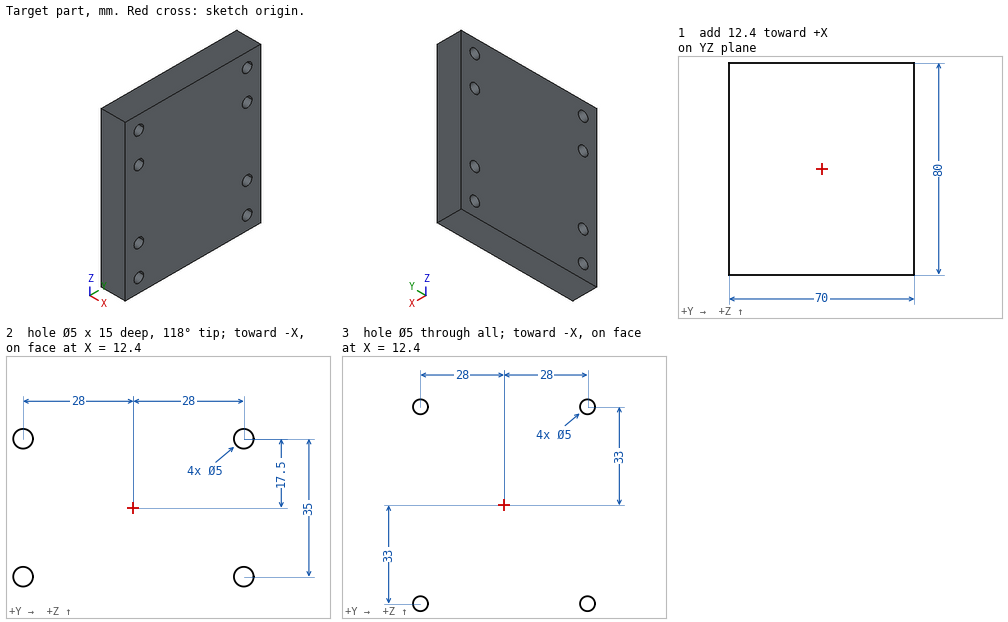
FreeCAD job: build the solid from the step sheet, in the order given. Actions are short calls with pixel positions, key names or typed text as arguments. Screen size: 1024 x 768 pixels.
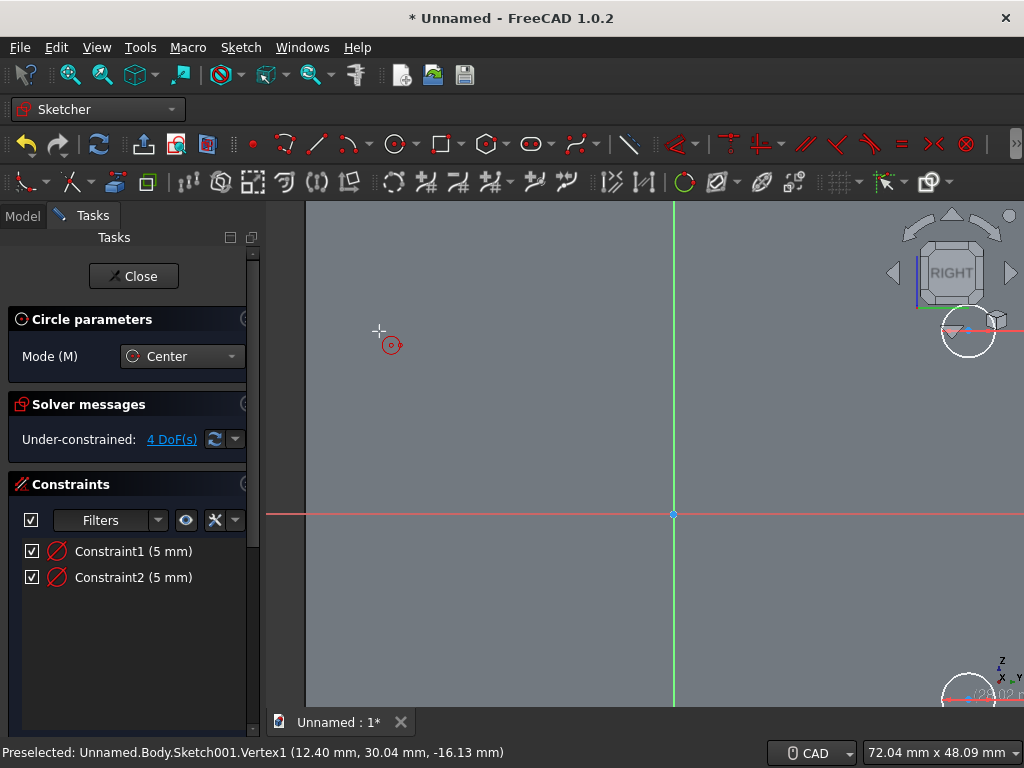
click(379, 330)
move(398, 312)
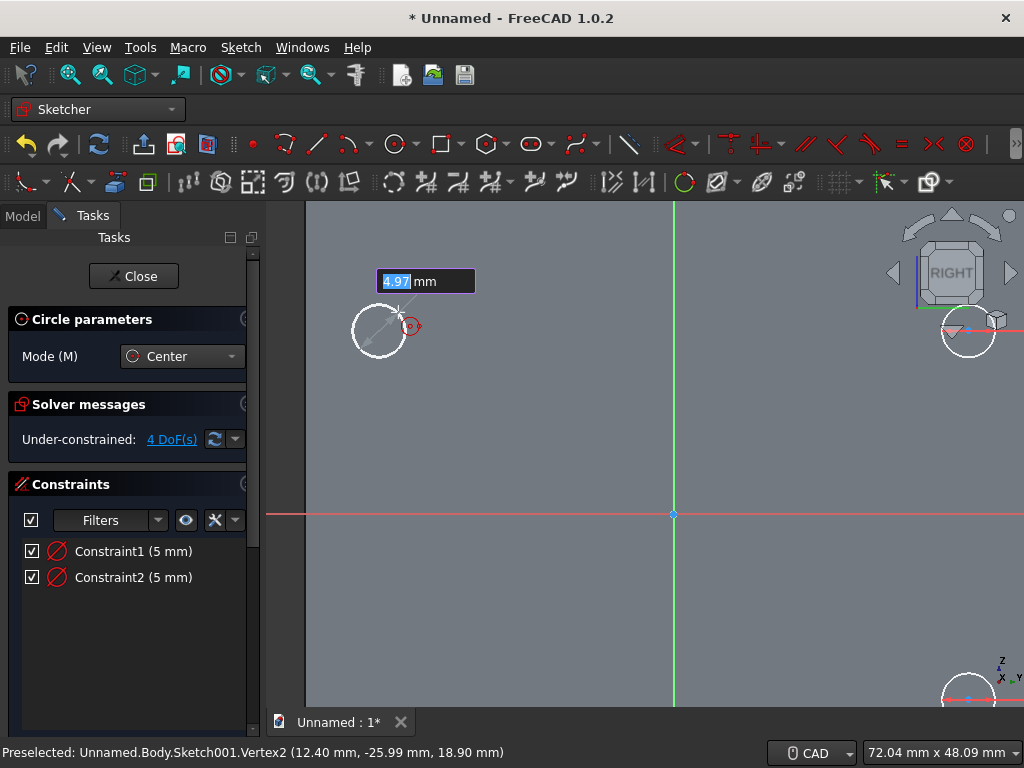
text(5)
key(Return)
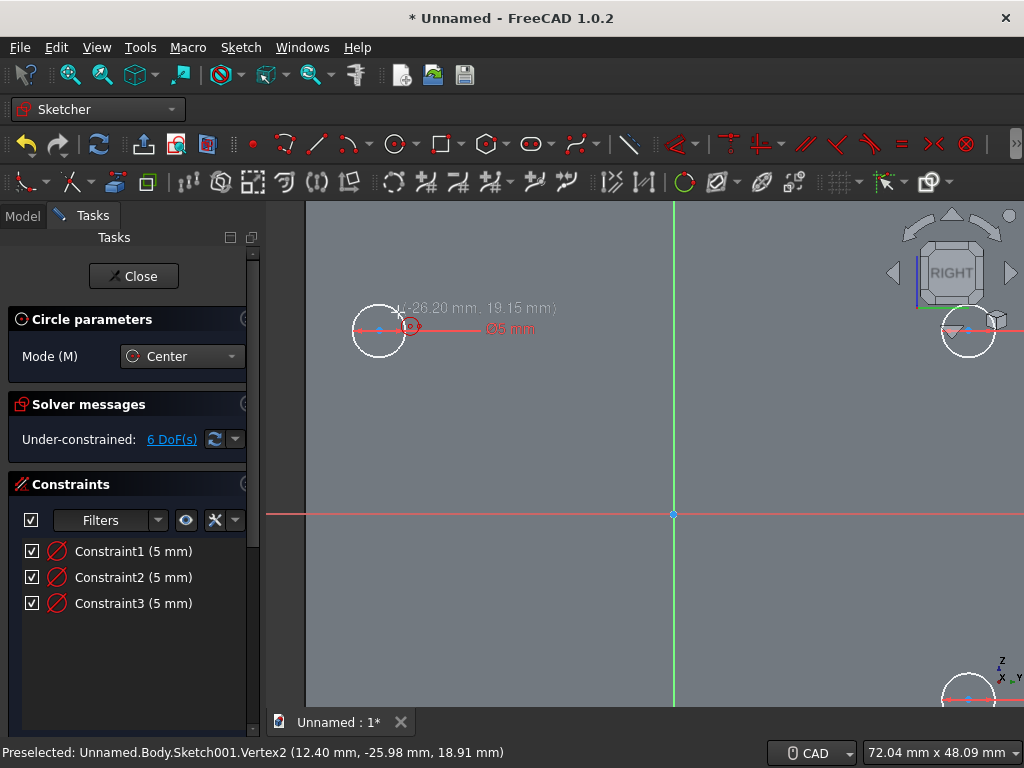
scroll(379, 331, down, 2)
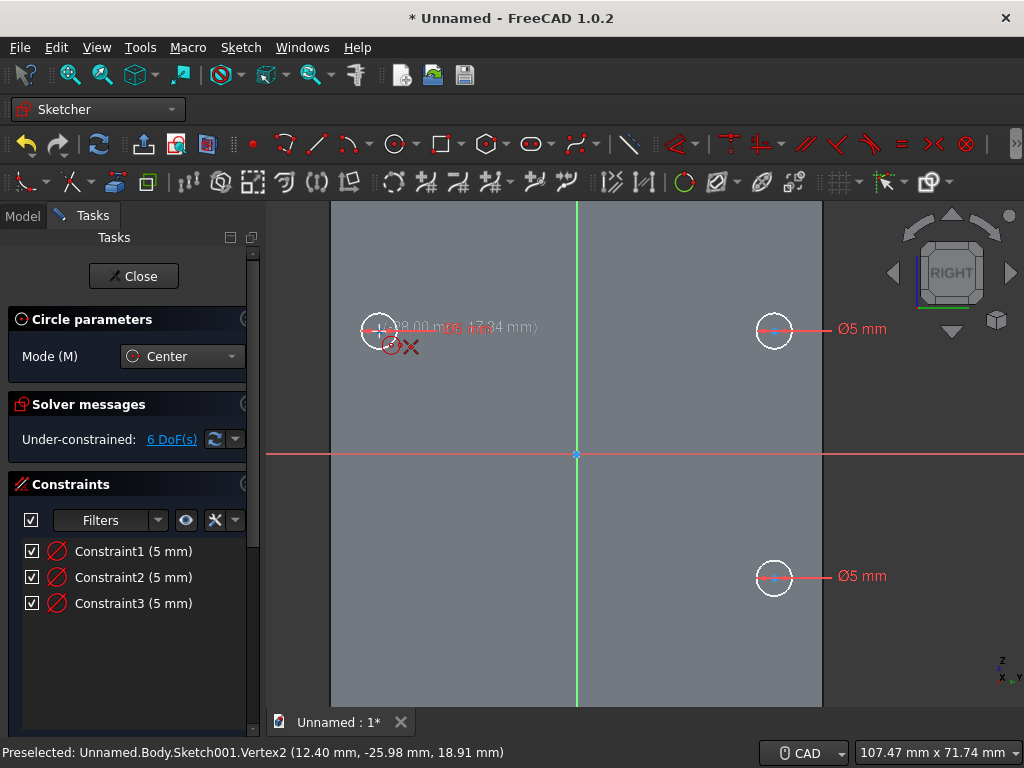
scroll(379, 578, up, 2)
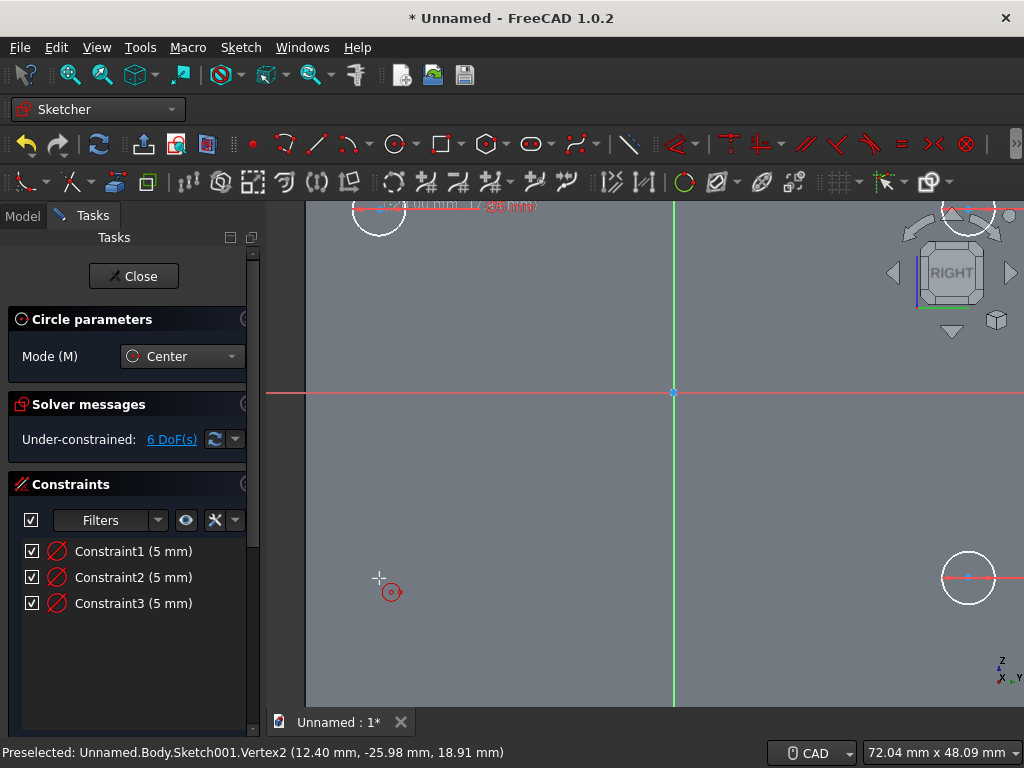
click(379, 577)
move(398, 558)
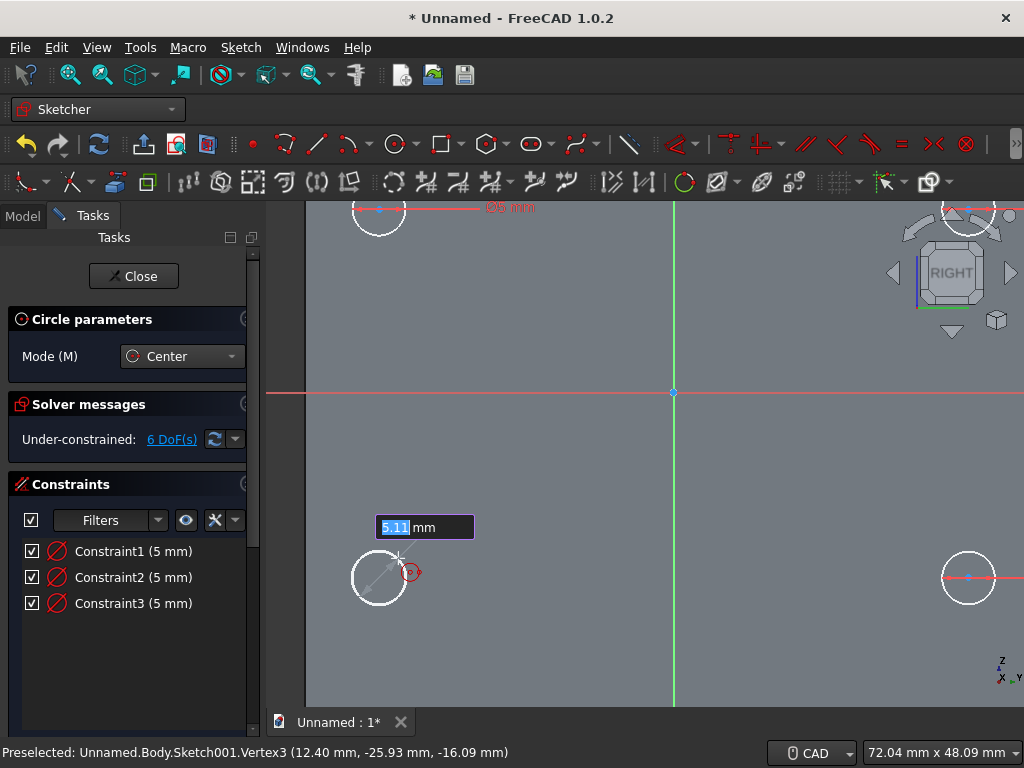
text(5)
key(Return)
key(Escape)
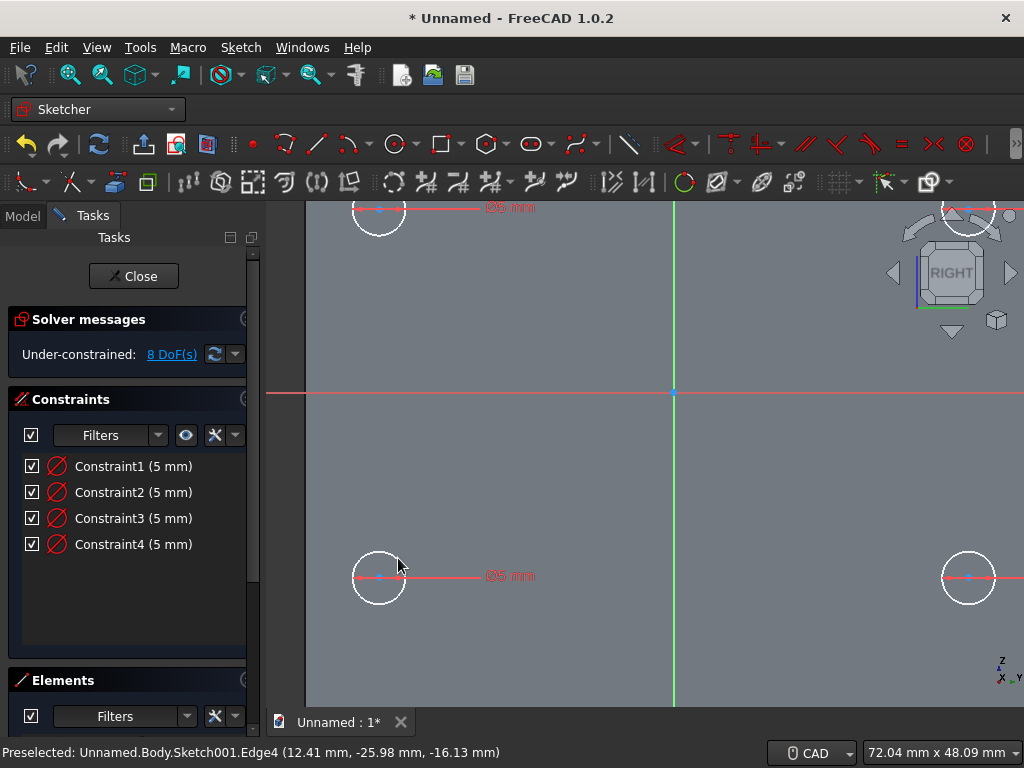
scroll(379, 578, down, 2)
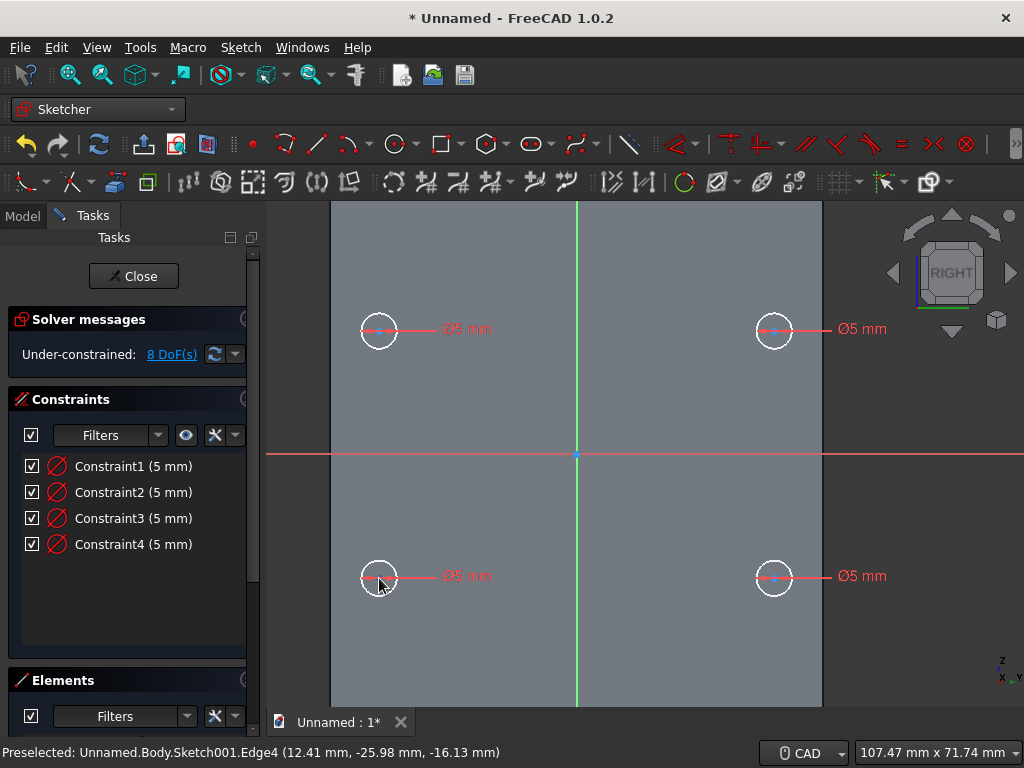
click(774, 331)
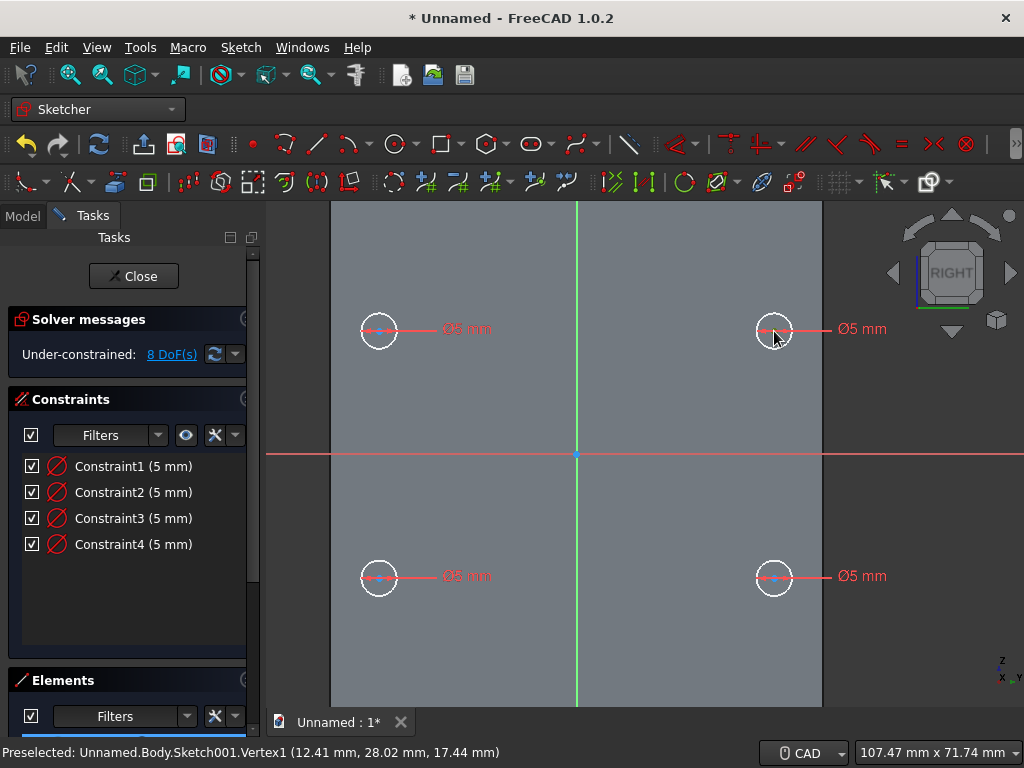
click(774, 578)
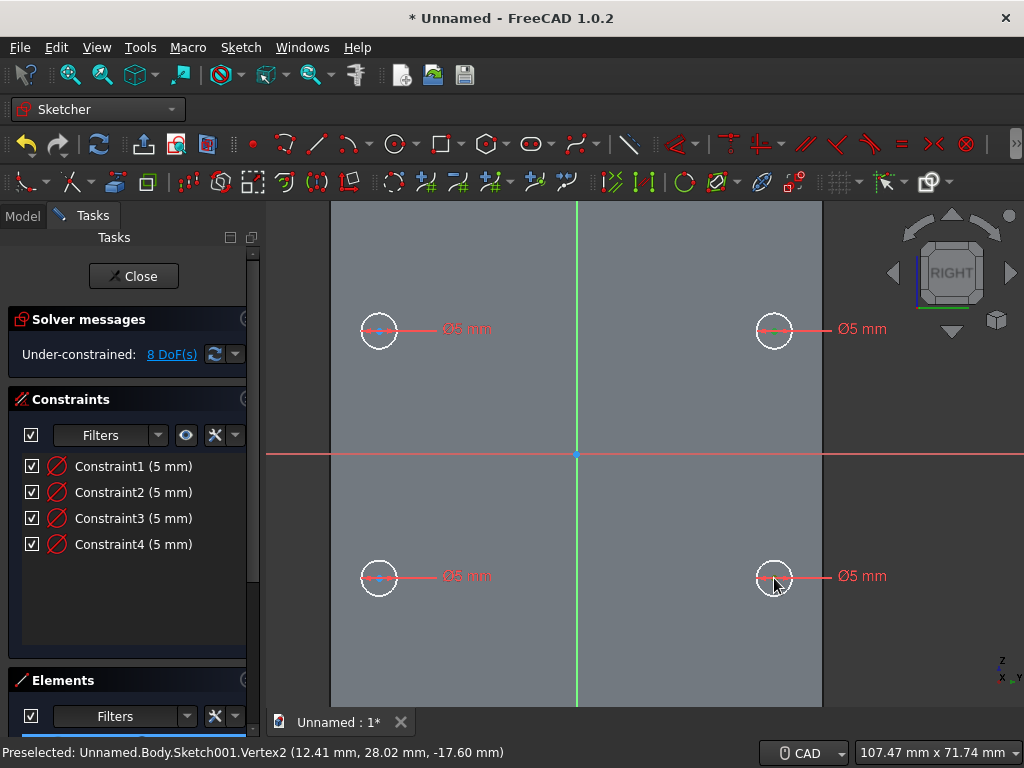
click(784, 144)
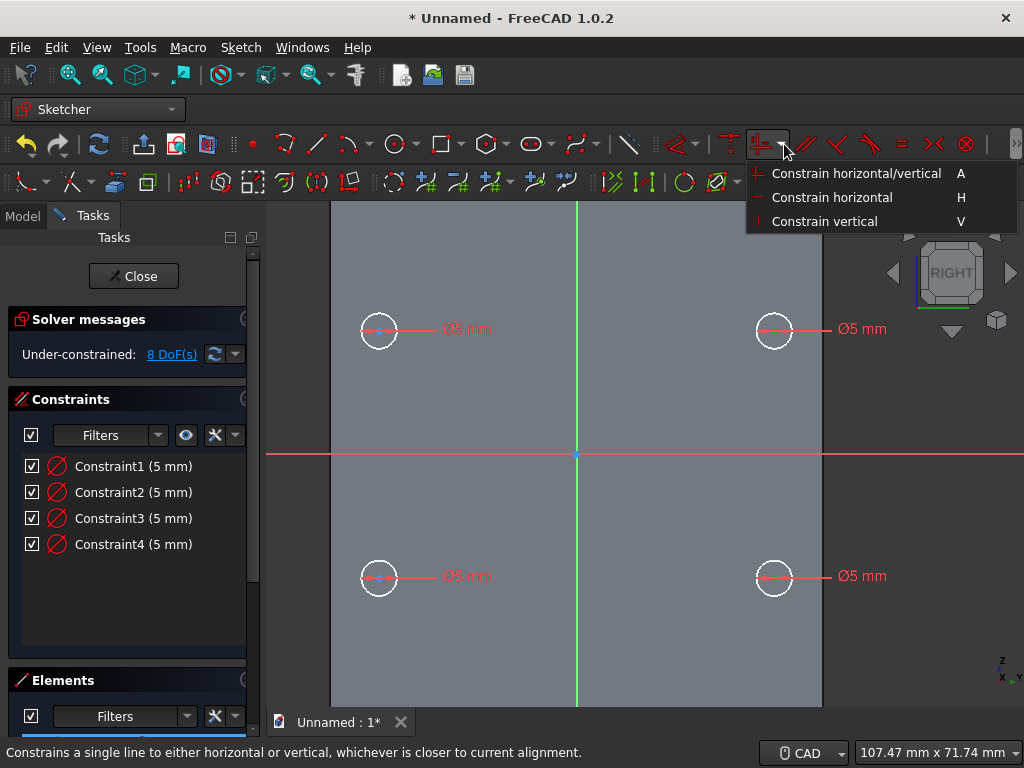
click(882, 221)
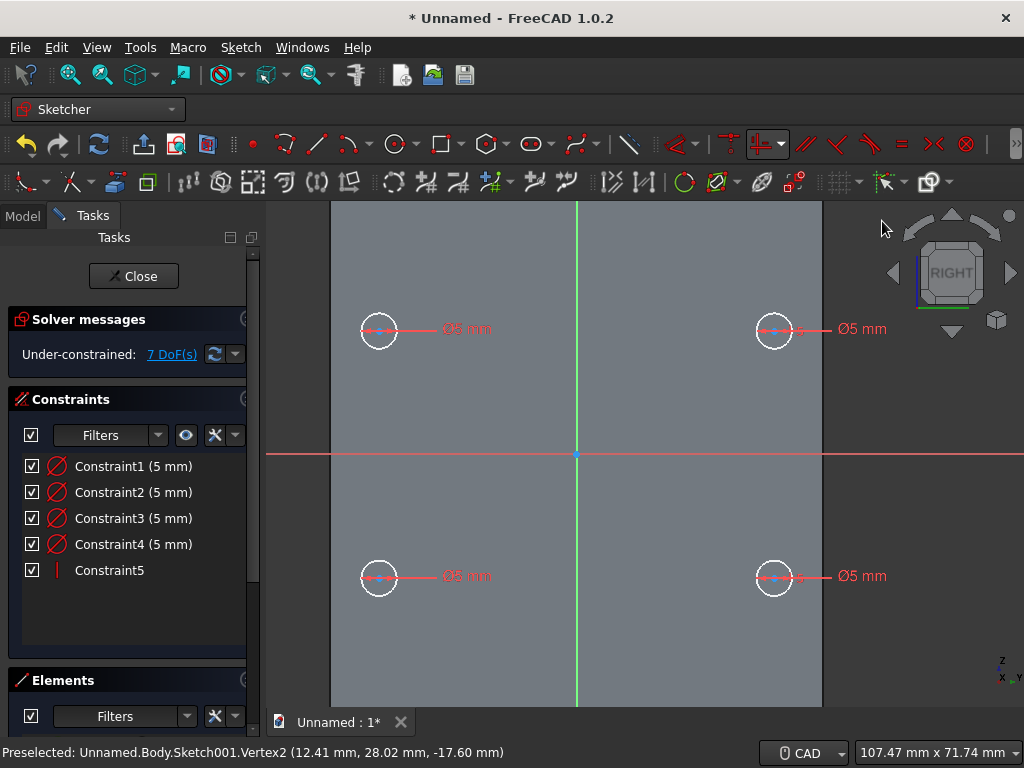
click(774, 331)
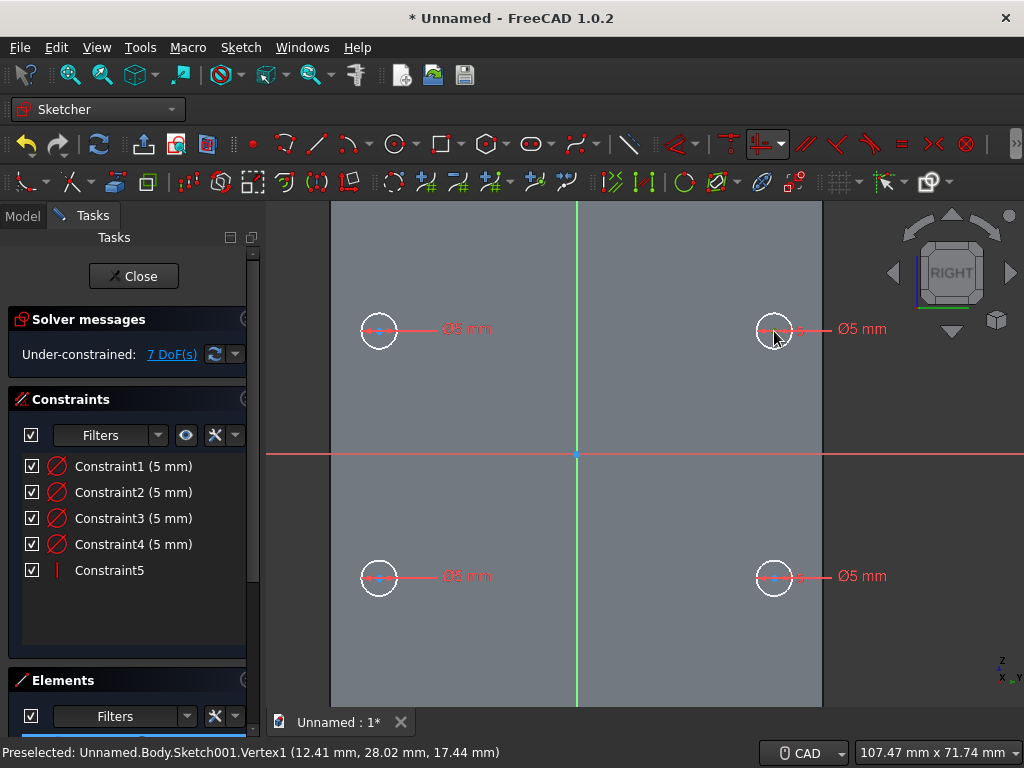
click(379, 331)